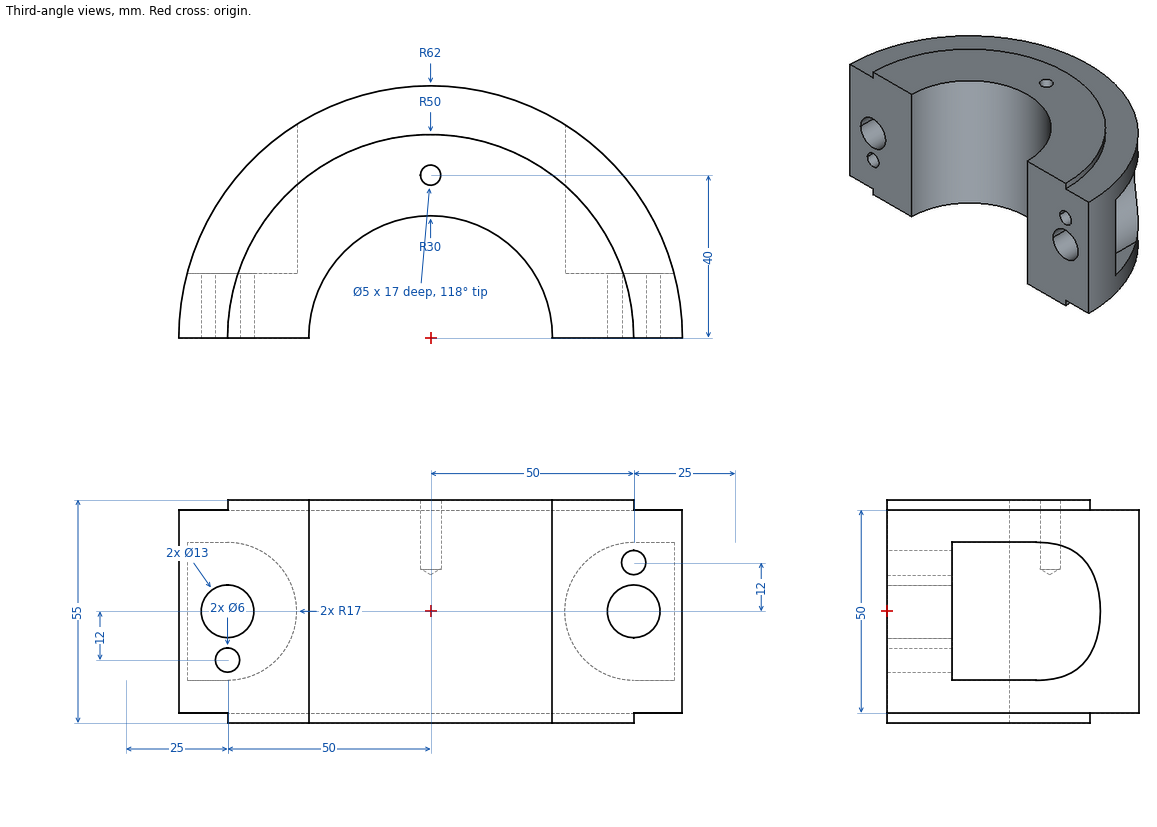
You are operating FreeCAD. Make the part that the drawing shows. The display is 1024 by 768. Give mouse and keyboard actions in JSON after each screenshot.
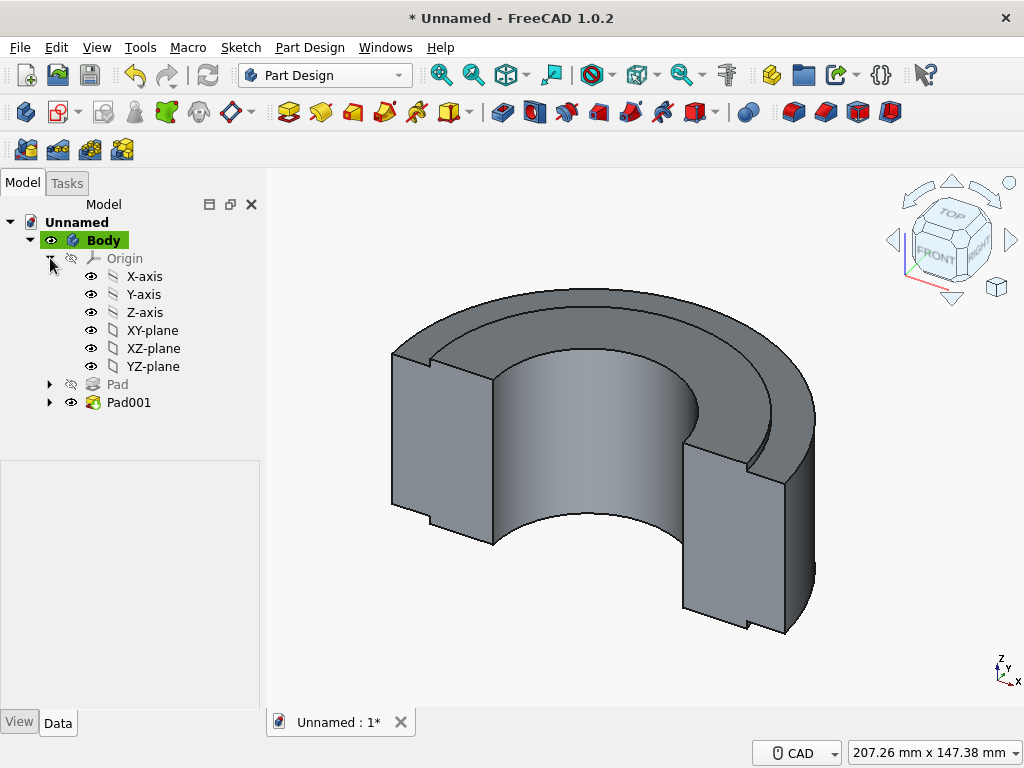
{"action": "left_click", "coordinate": [136, 348]}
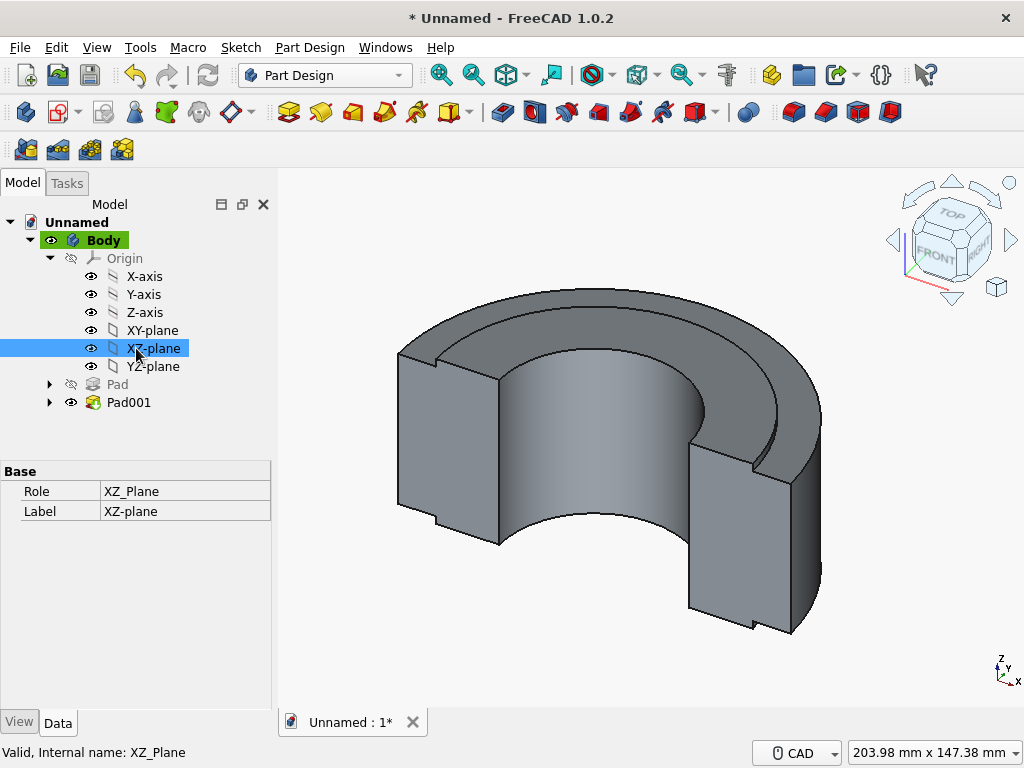
{"action": "left_click", "coordinate": [232, 112]}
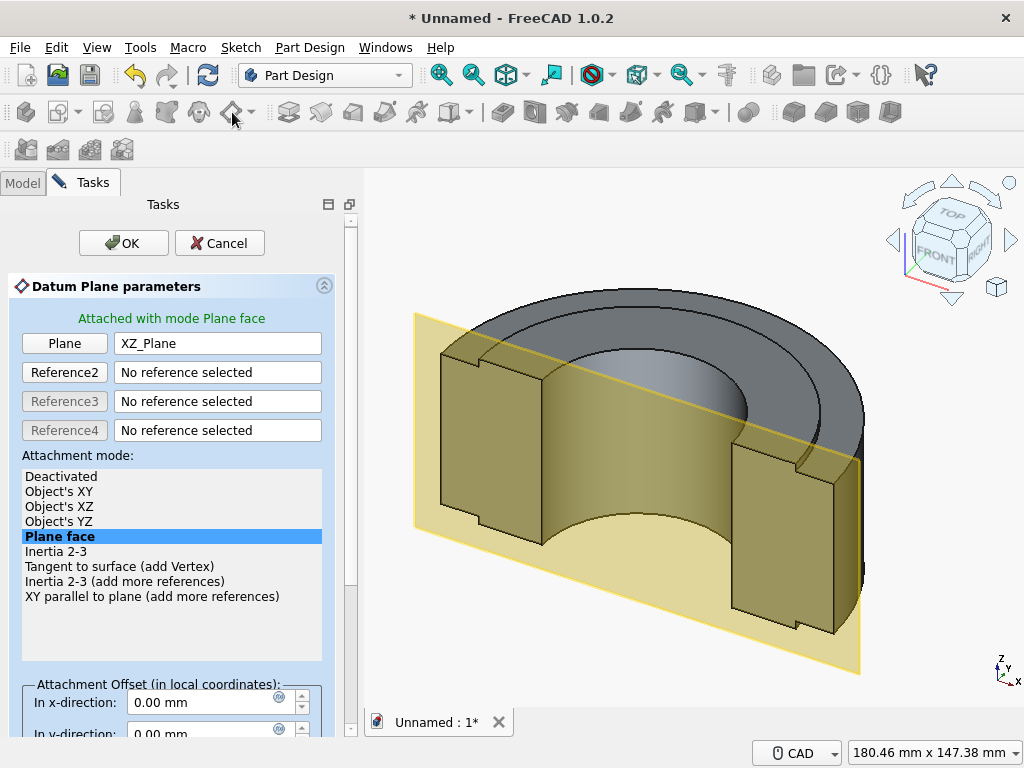
{"action": "scroll", "coordinate": [351, 475], "scroll_direction": "down", "scroll_amount": 2}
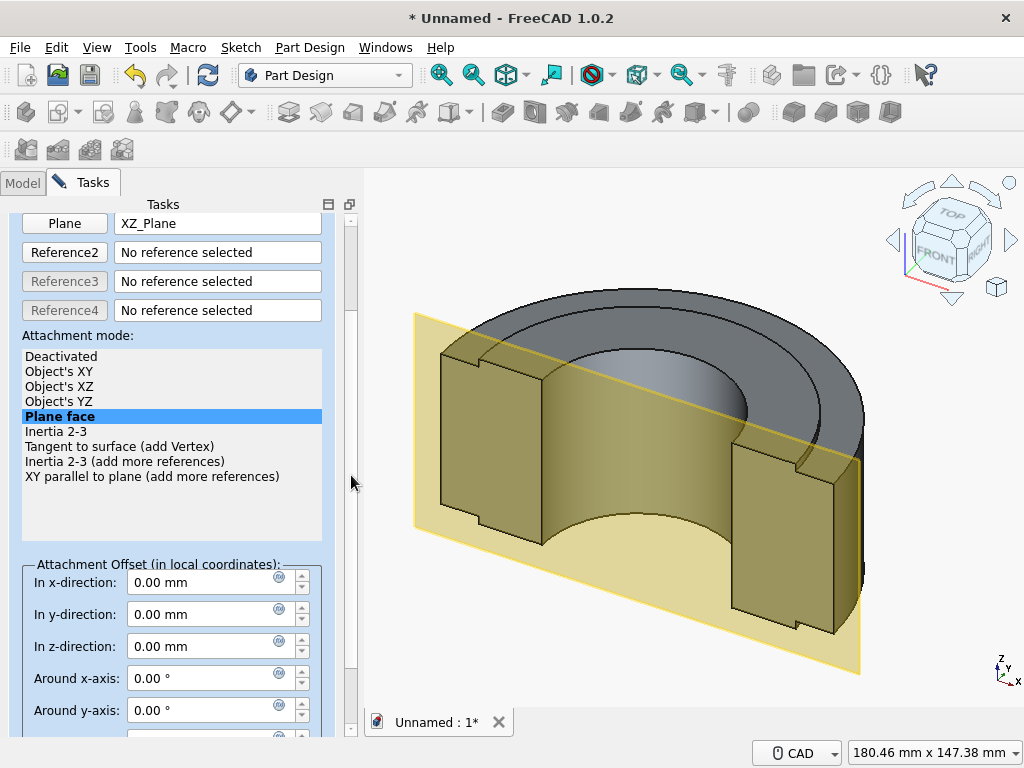
{"action": "triple_click", "coordinate": [210, 646]}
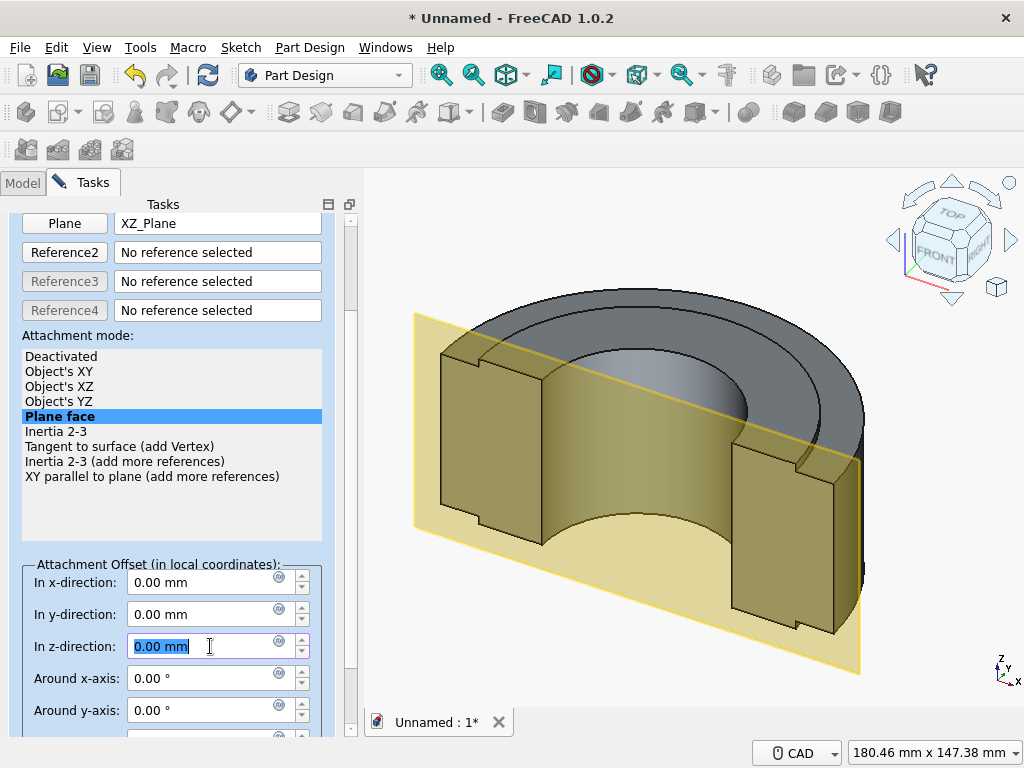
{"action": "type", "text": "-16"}
{"action": "key", "text": "Tab"}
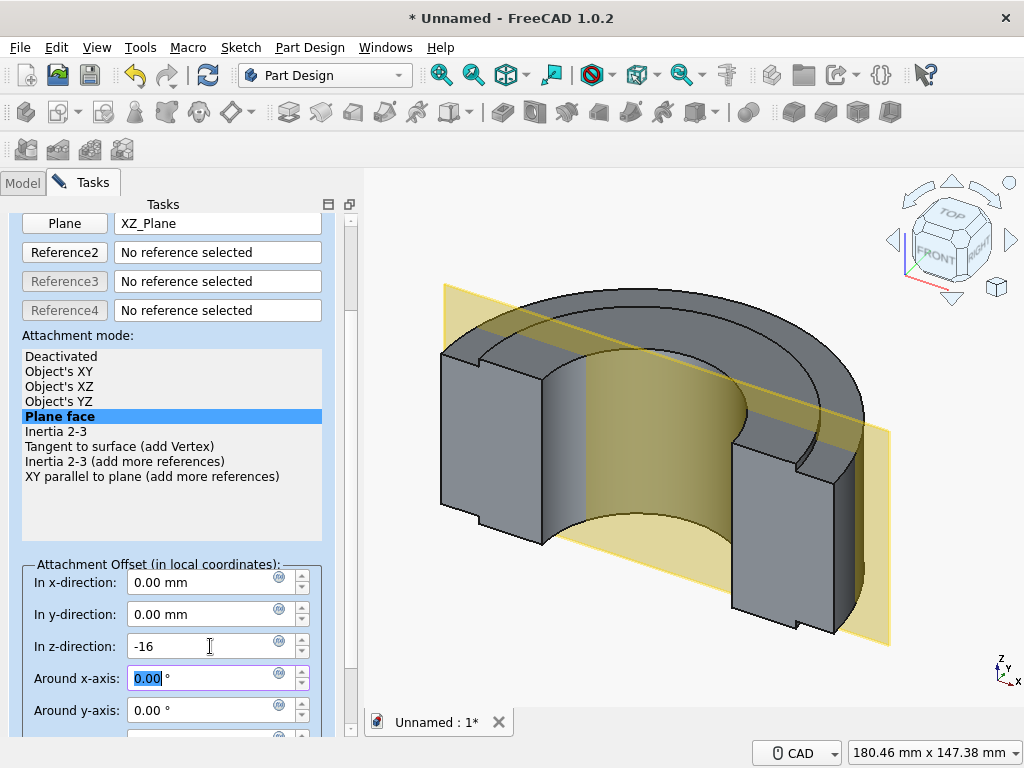
{"action": "scroll", "coordinate": [351, 475], "scroll_direction": "up", "scroll_amount": 3}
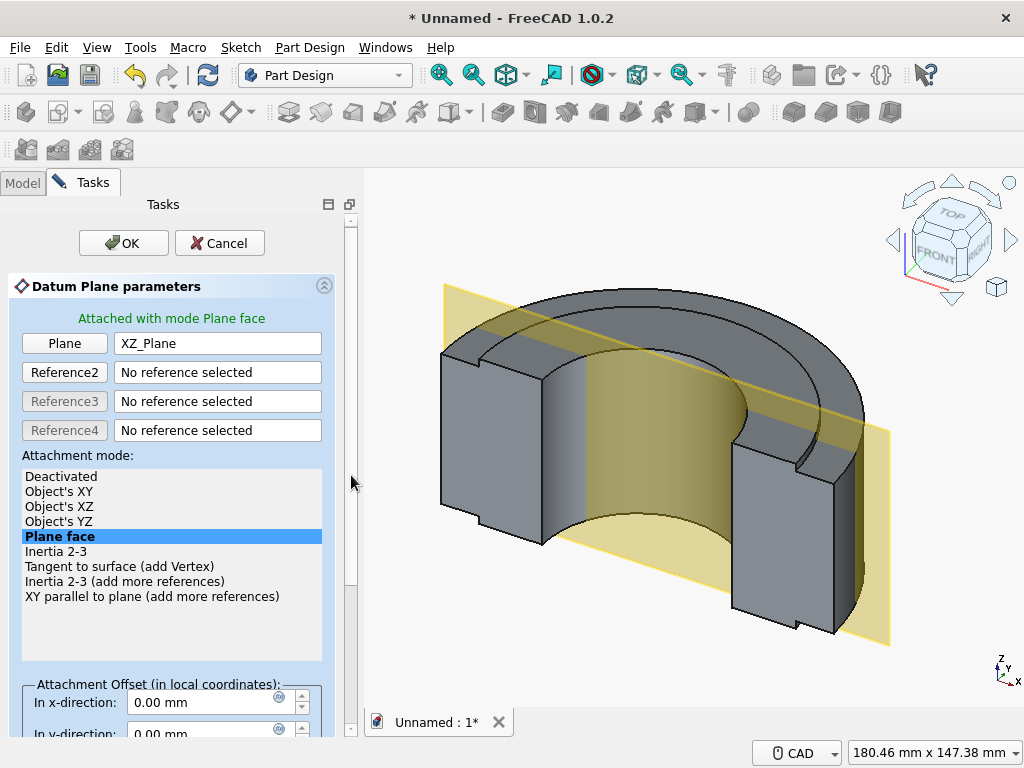
{"action": "left_click", "coordinate": [124, 243]}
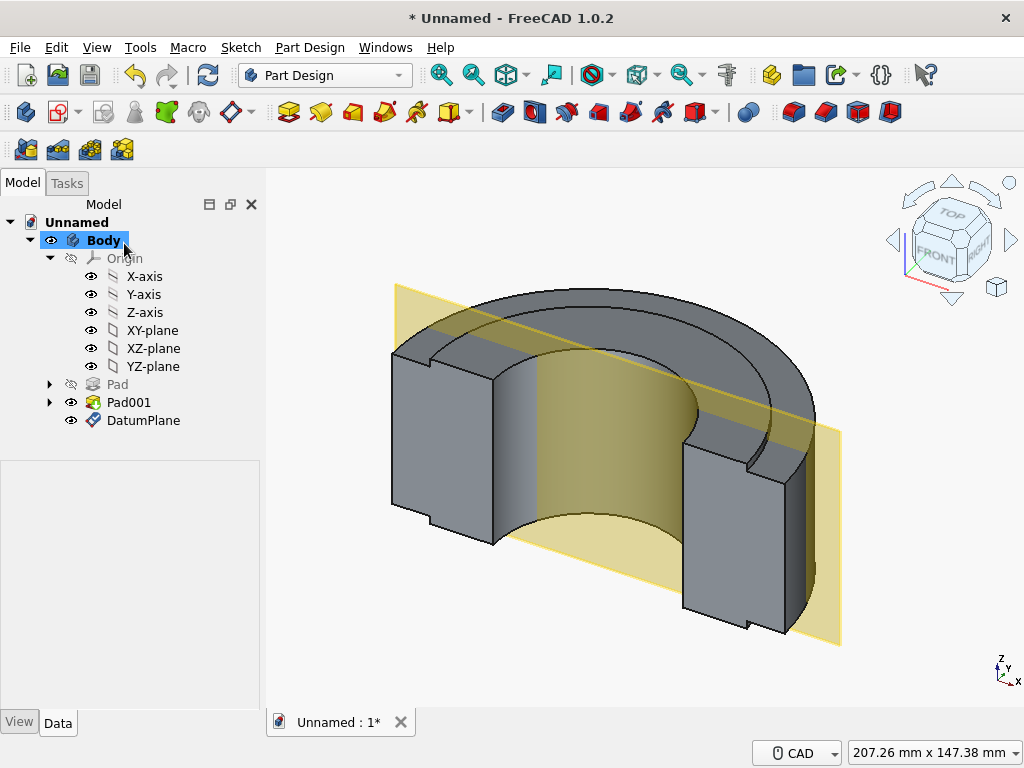
{"action": "left_click", "coordinate": [116, 420]}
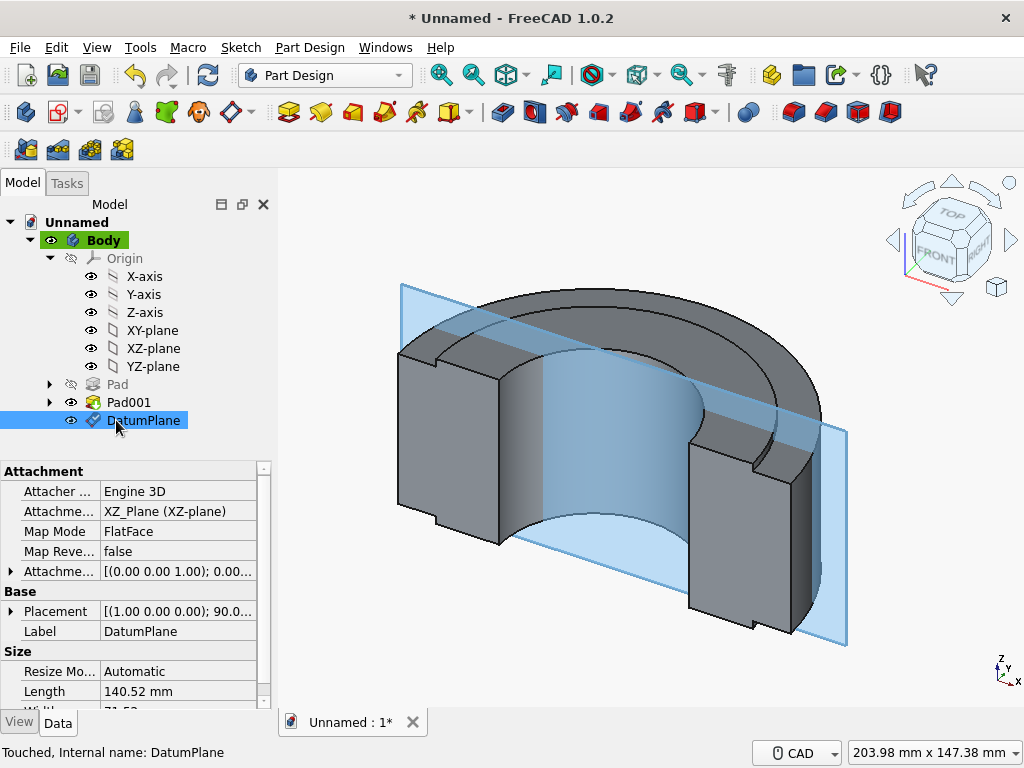
{"action": "left_click", "coordinate": [58, 112]}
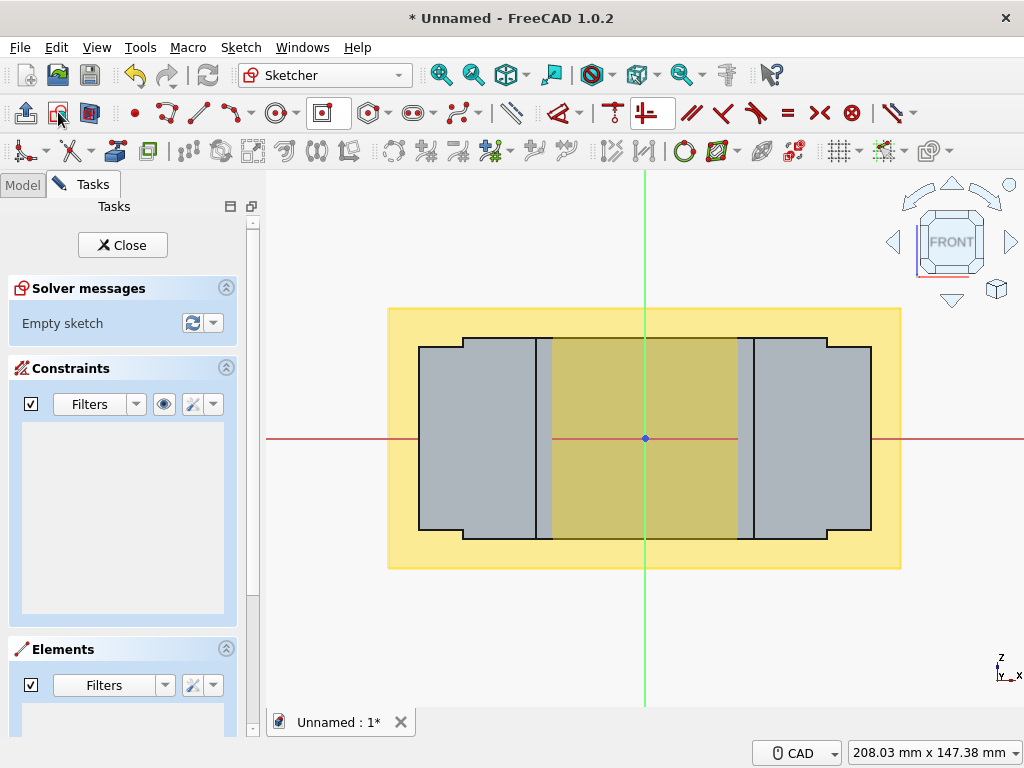
{"action": "left_click", "coordinate": [90, 114]}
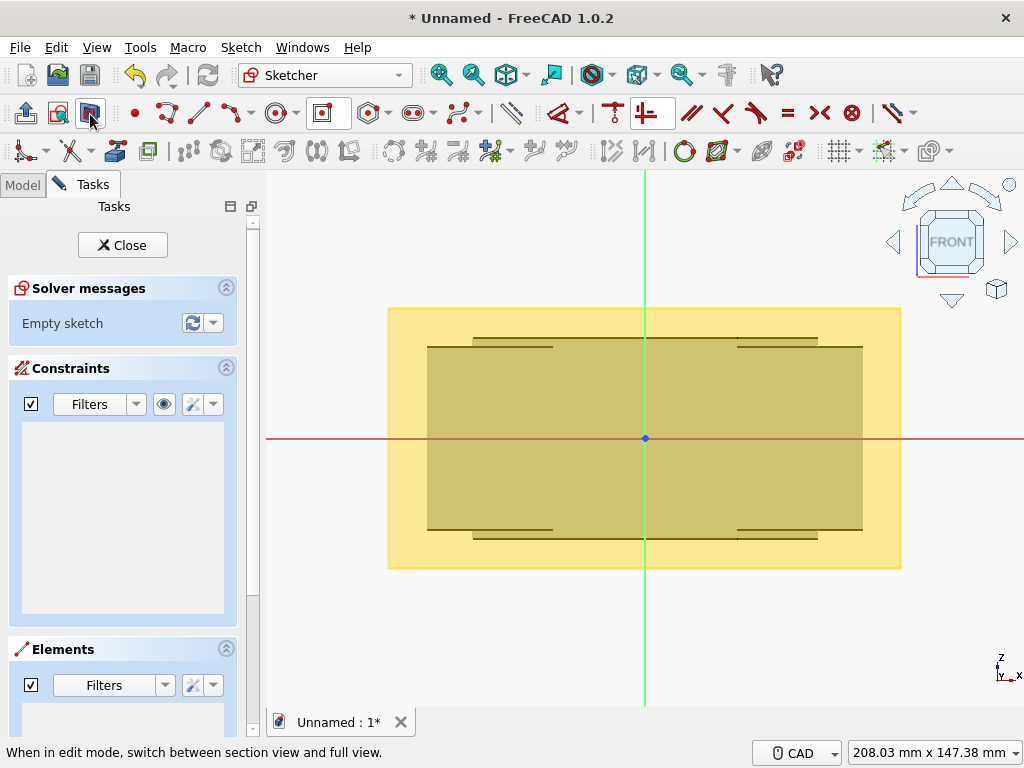
{"action": "scroll", "coordinate": [437, 438], "scroll_direction": "down", "scroll_amount": 2}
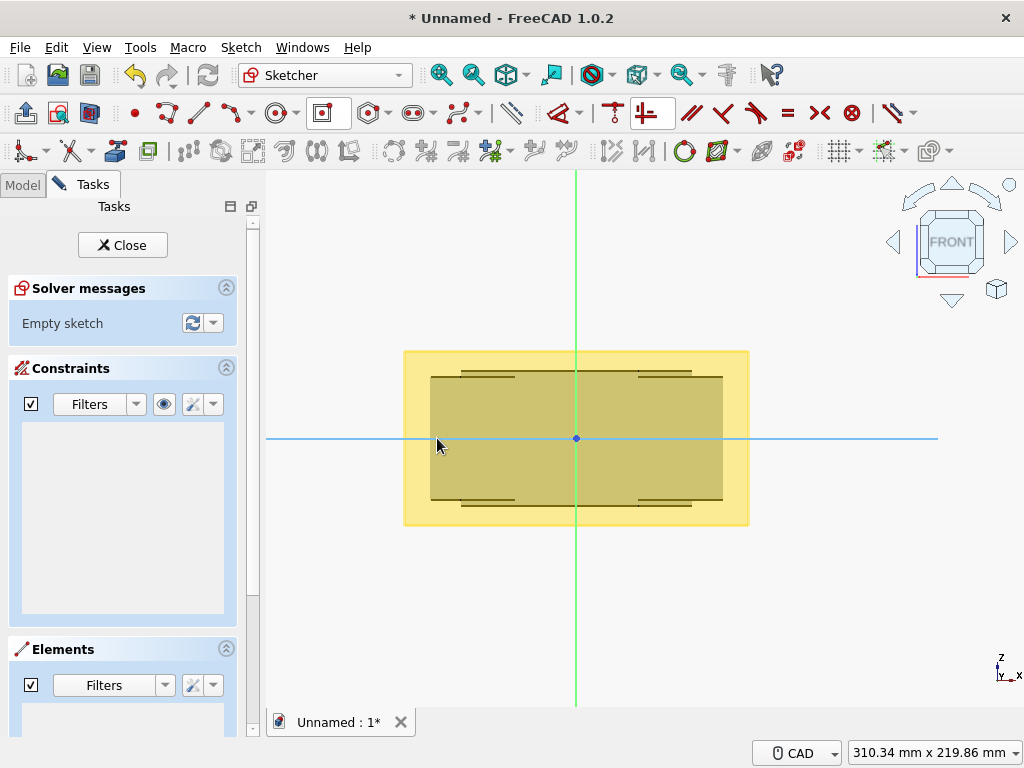
{"action": "left_click", "coordinate": [168, 114]}